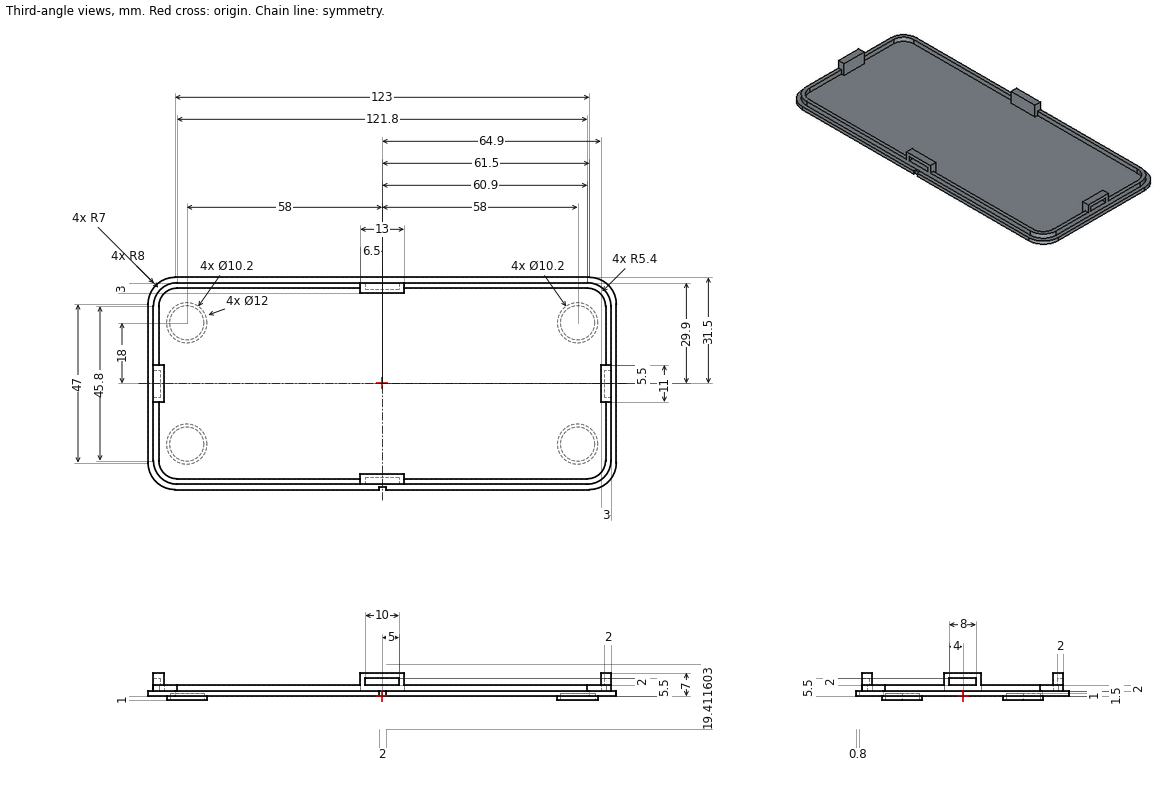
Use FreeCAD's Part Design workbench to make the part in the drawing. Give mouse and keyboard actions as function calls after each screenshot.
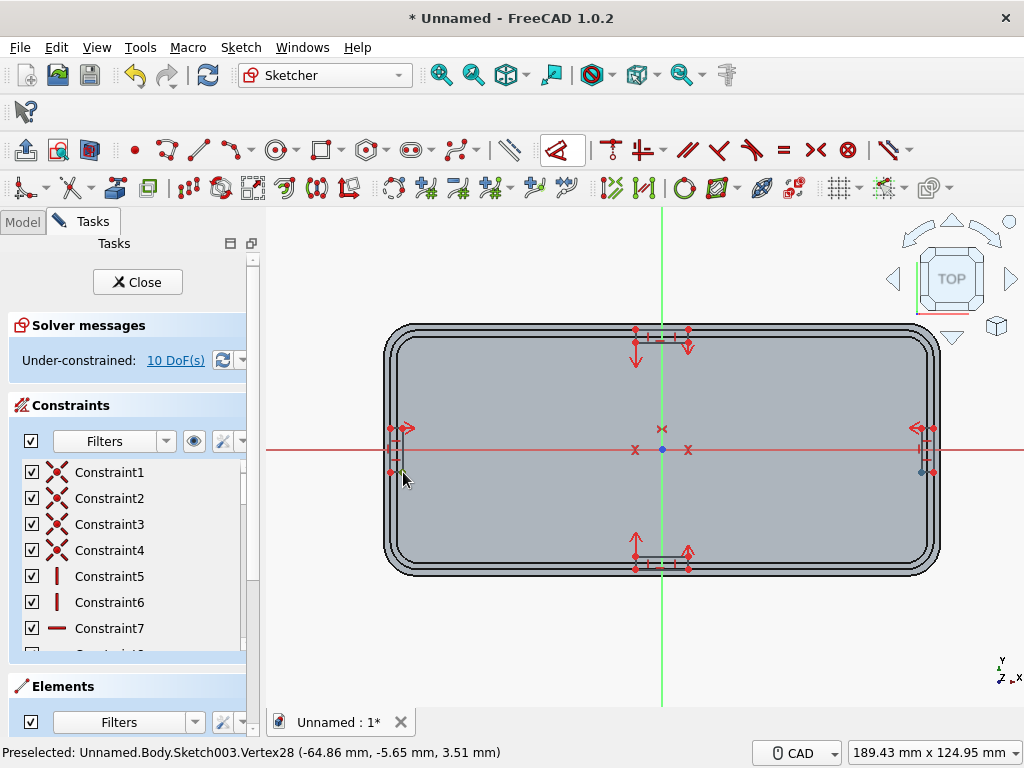
click(662, 647)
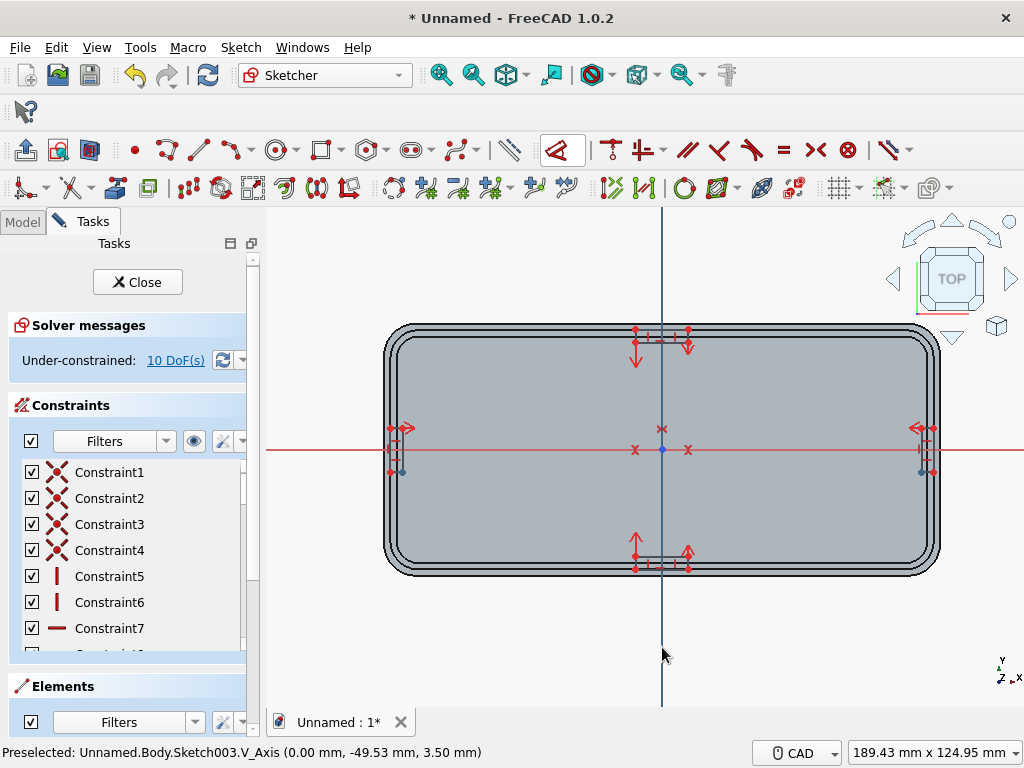
key(s)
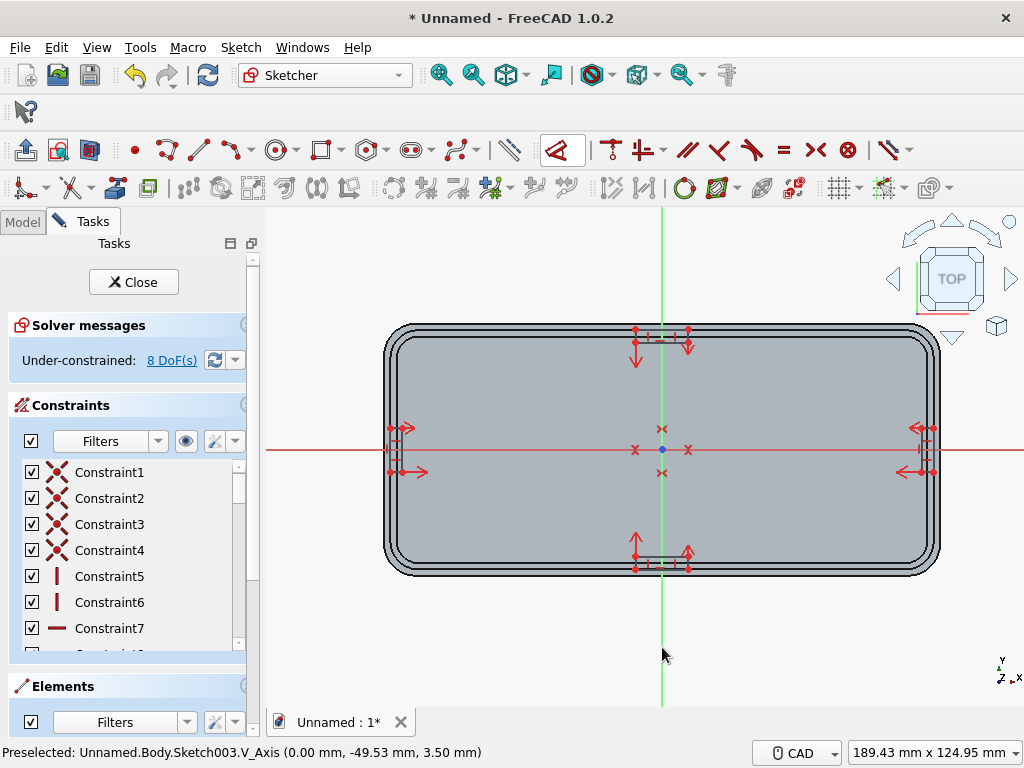
scroll(636, 336, up, 6)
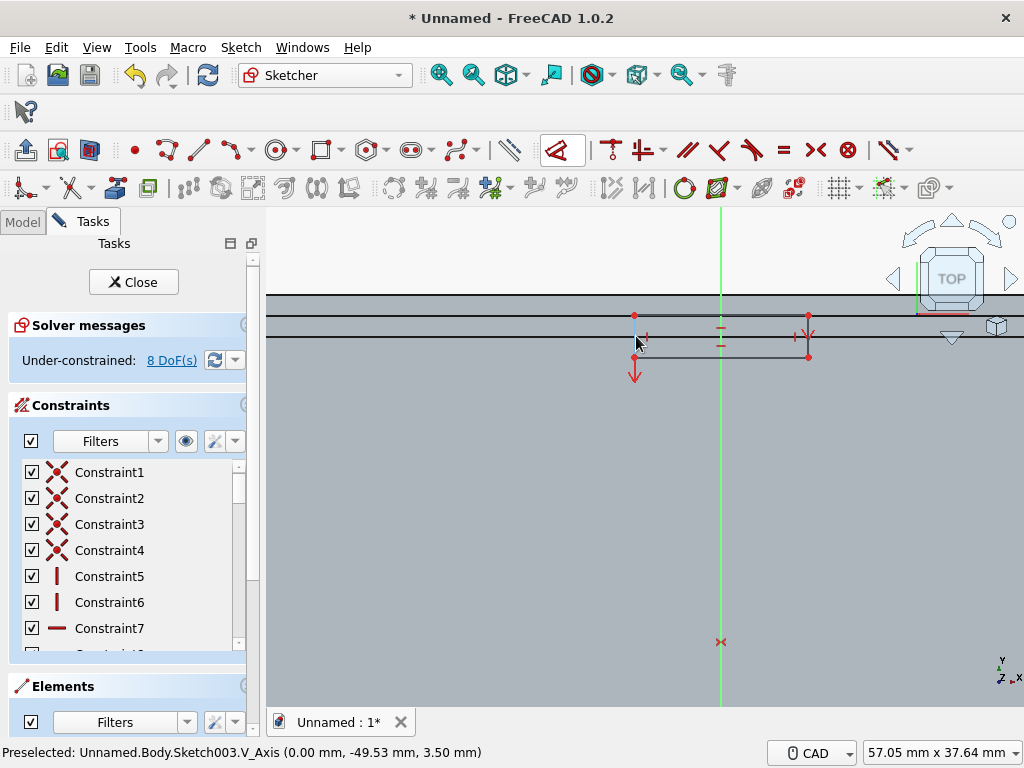
click(635, 336)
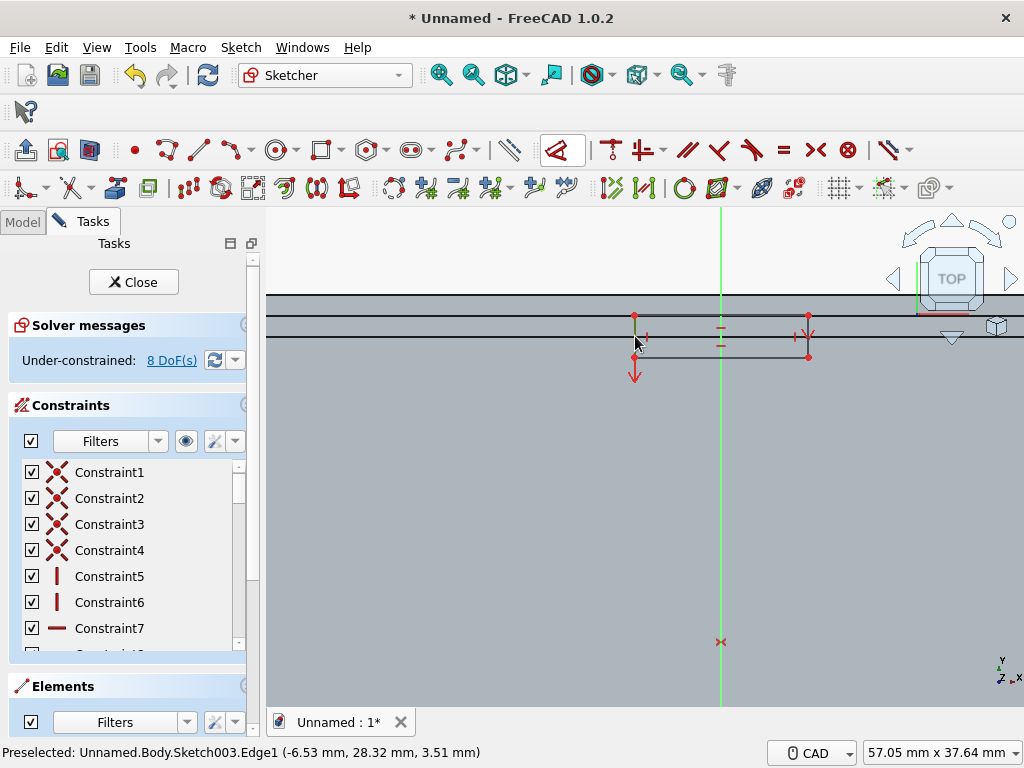
key(i)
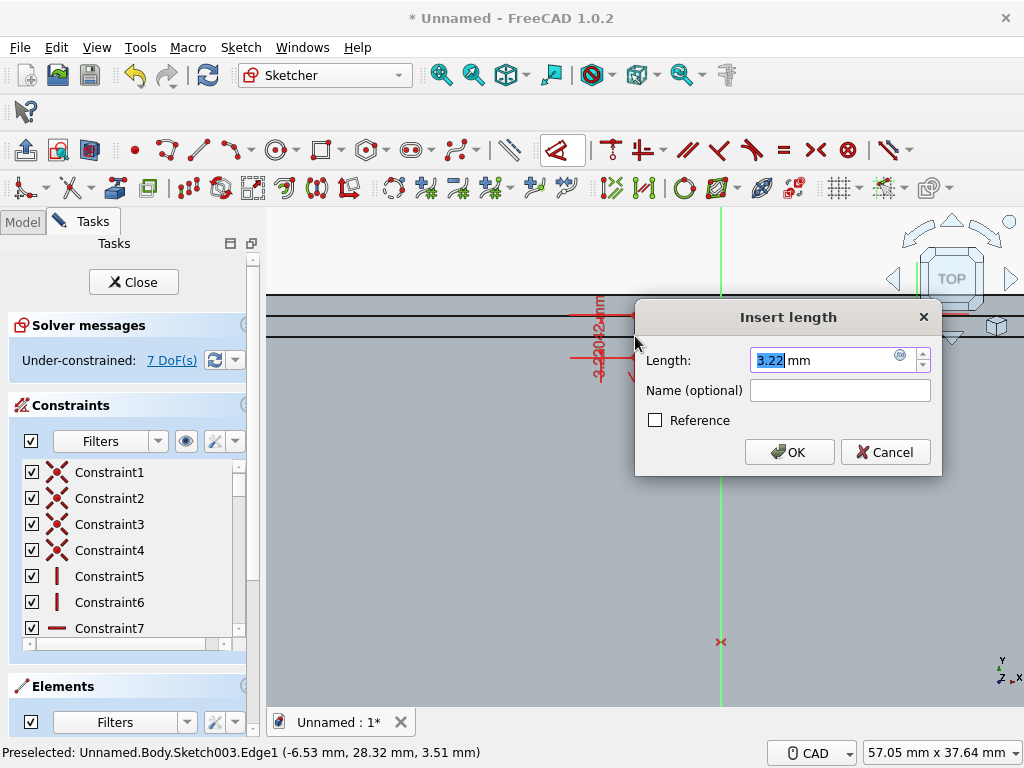
text(3)
key(Return)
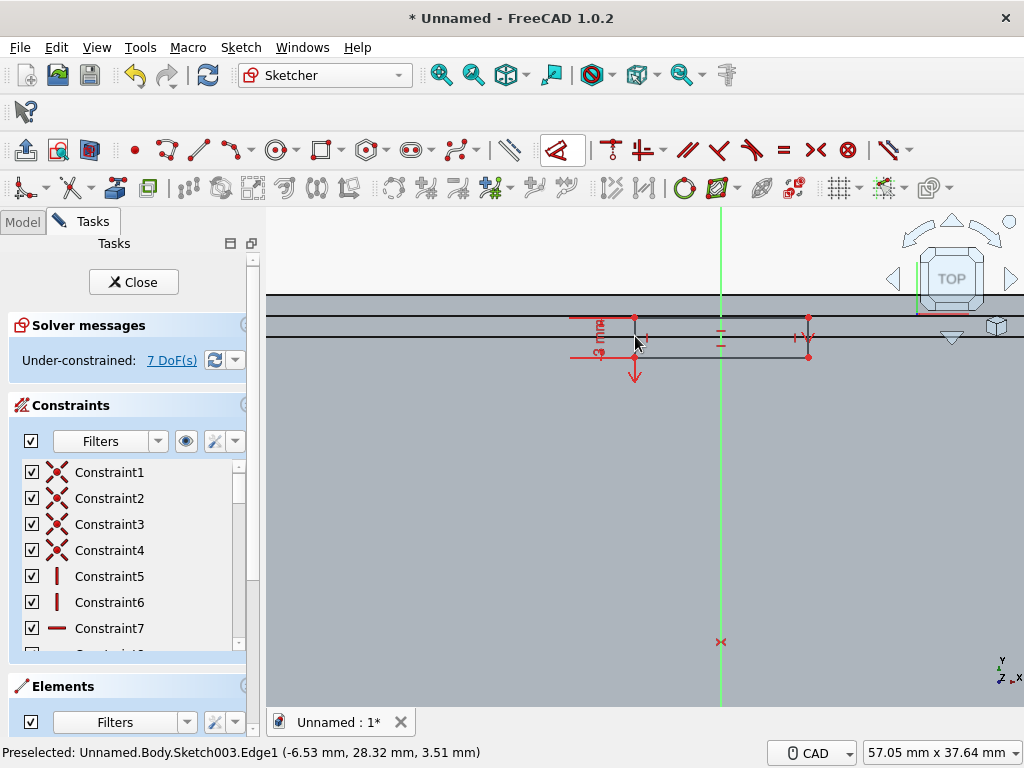
scroll(540, 392, down, 8)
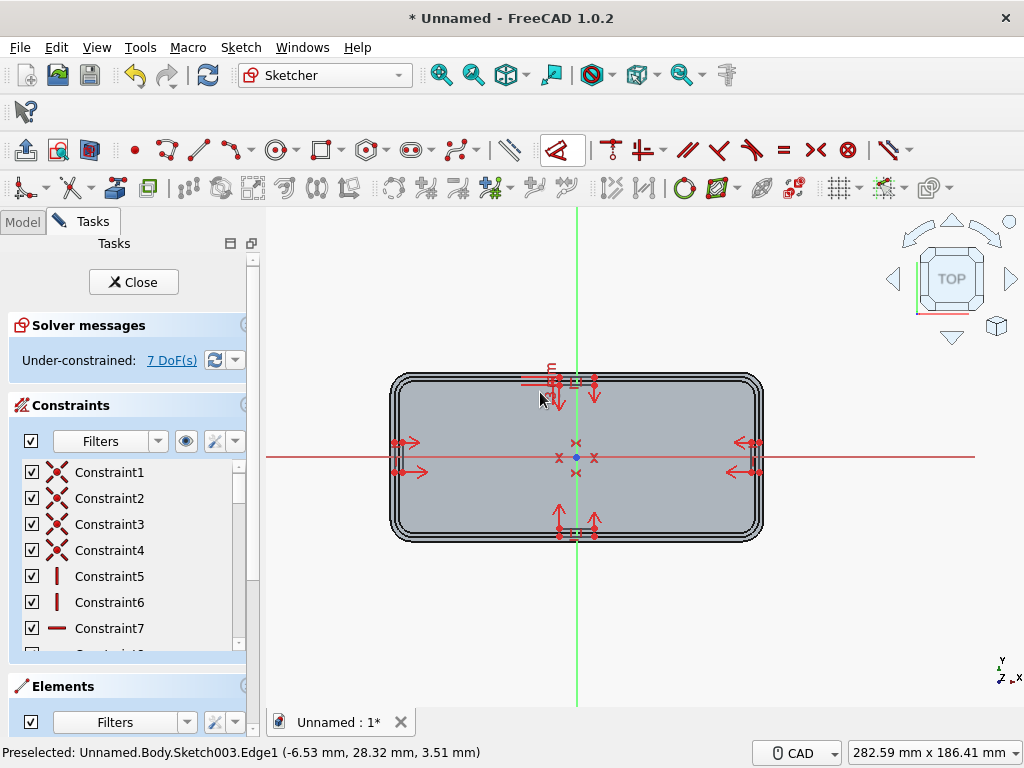
scroll(754, 472, up, 9)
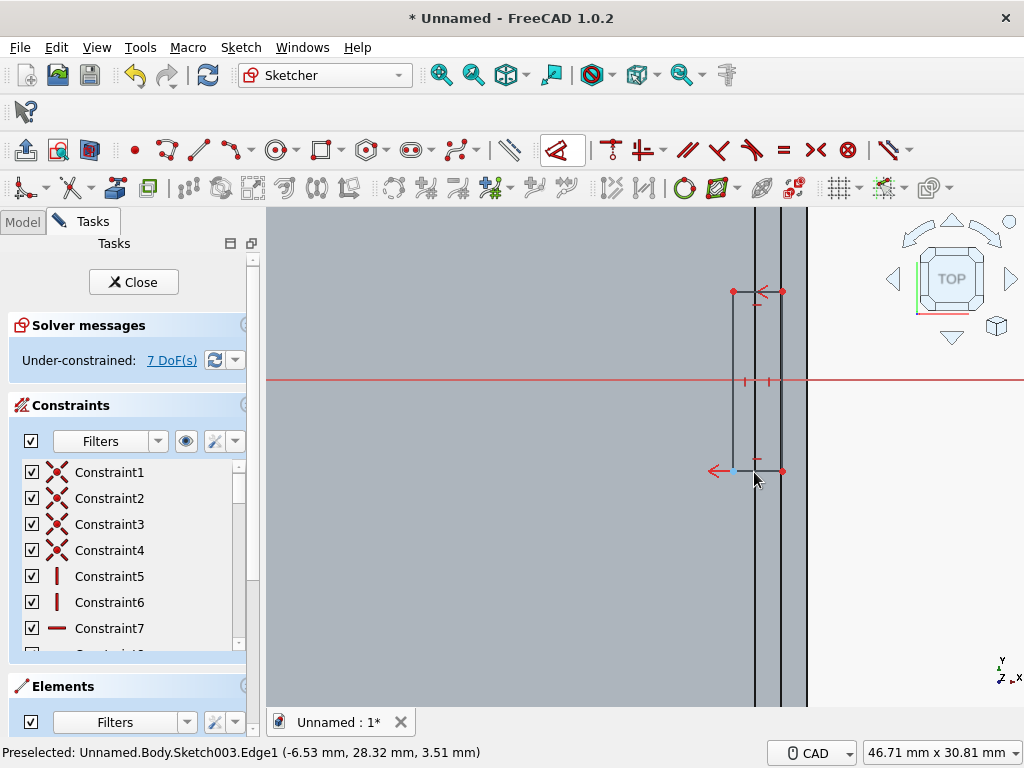
click(748, 471)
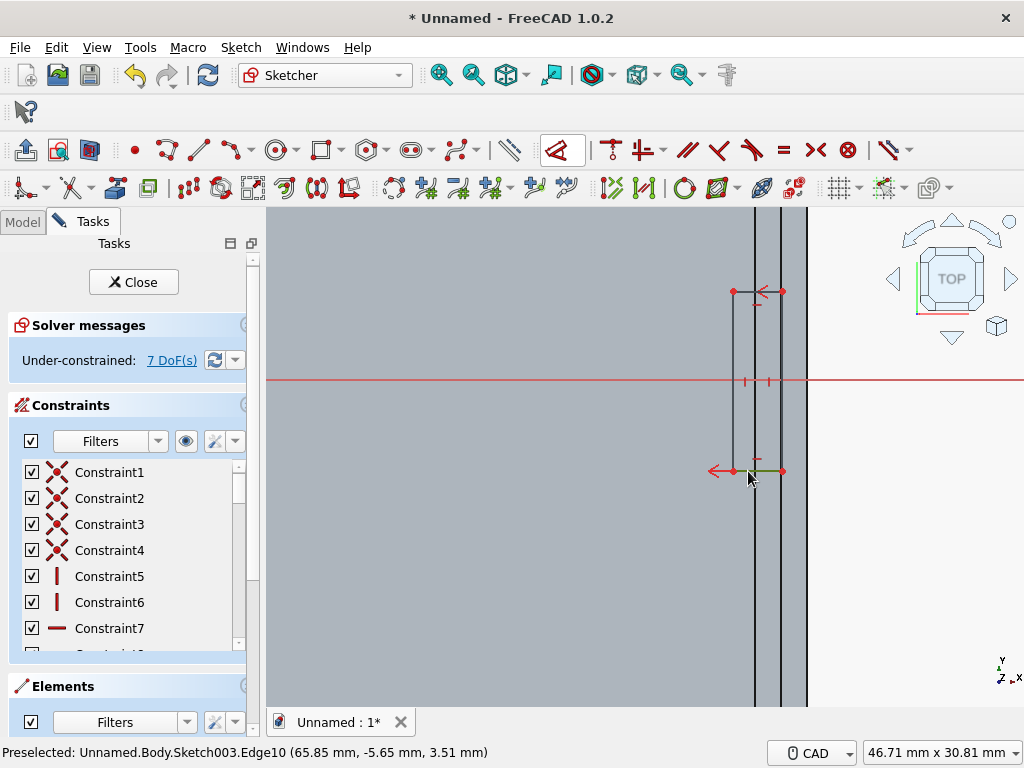
key(l)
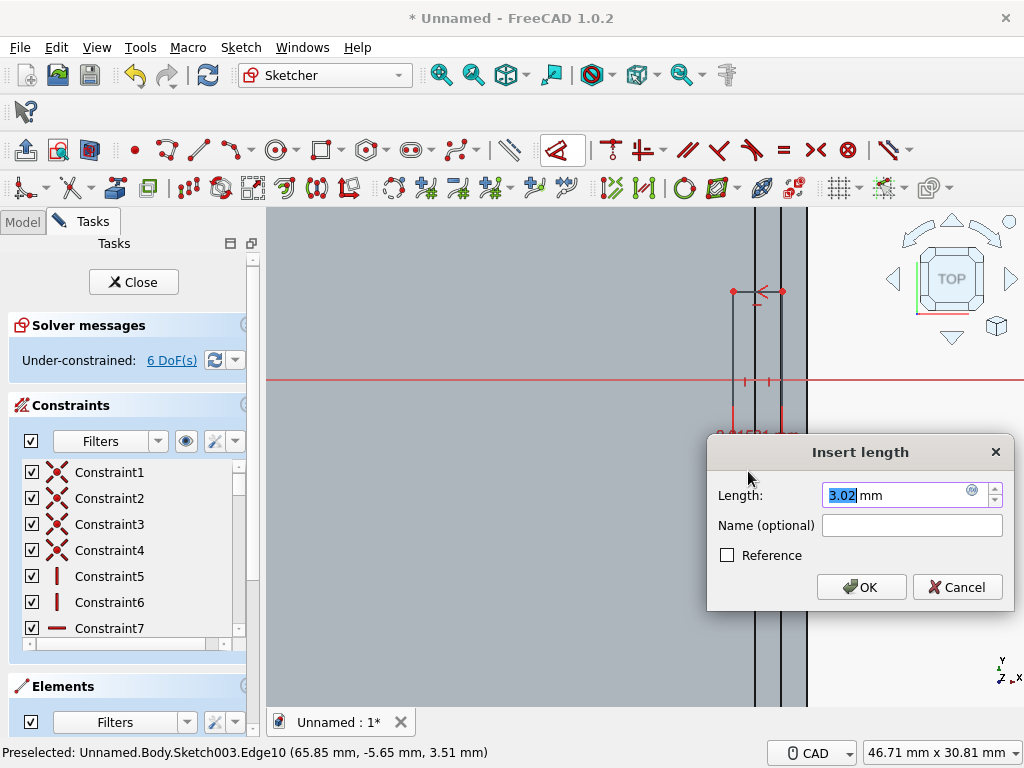
text(3)
key(Return)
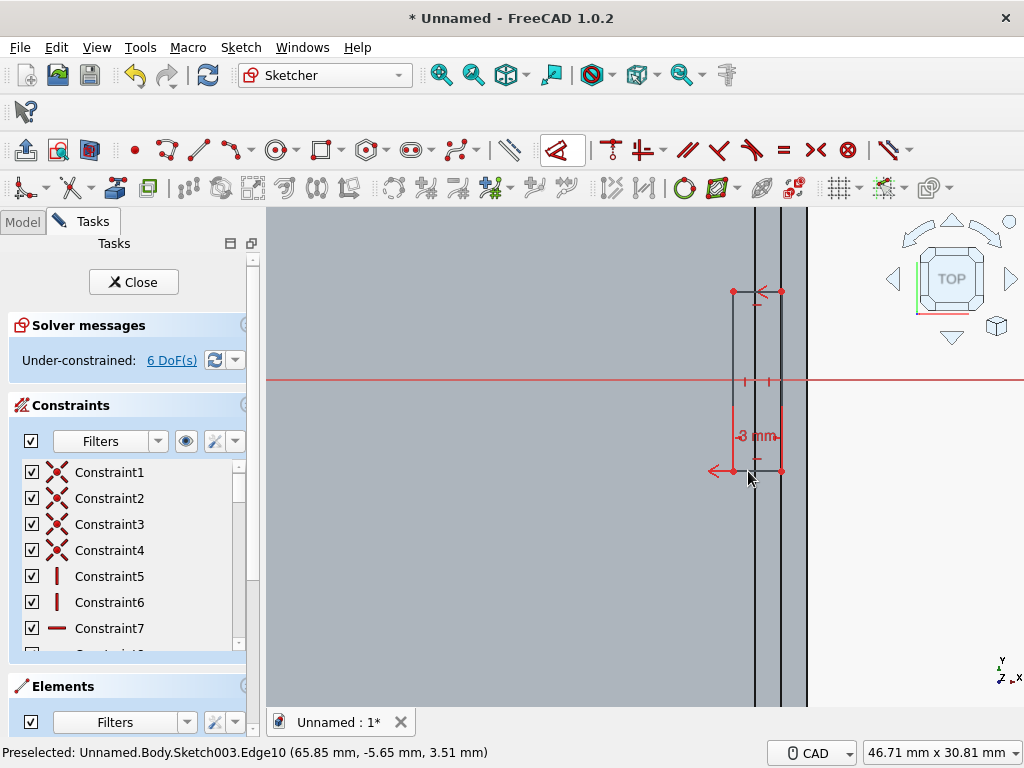
scroll(754, 472, down, 9)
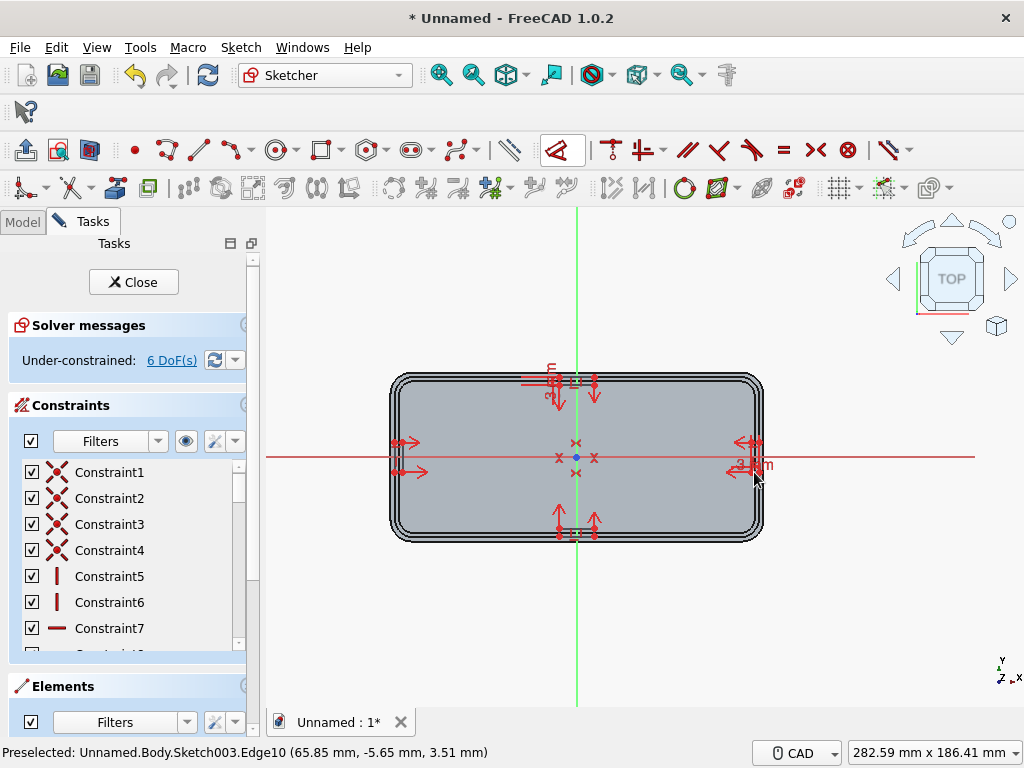
scroll(570, 385, up, 4)